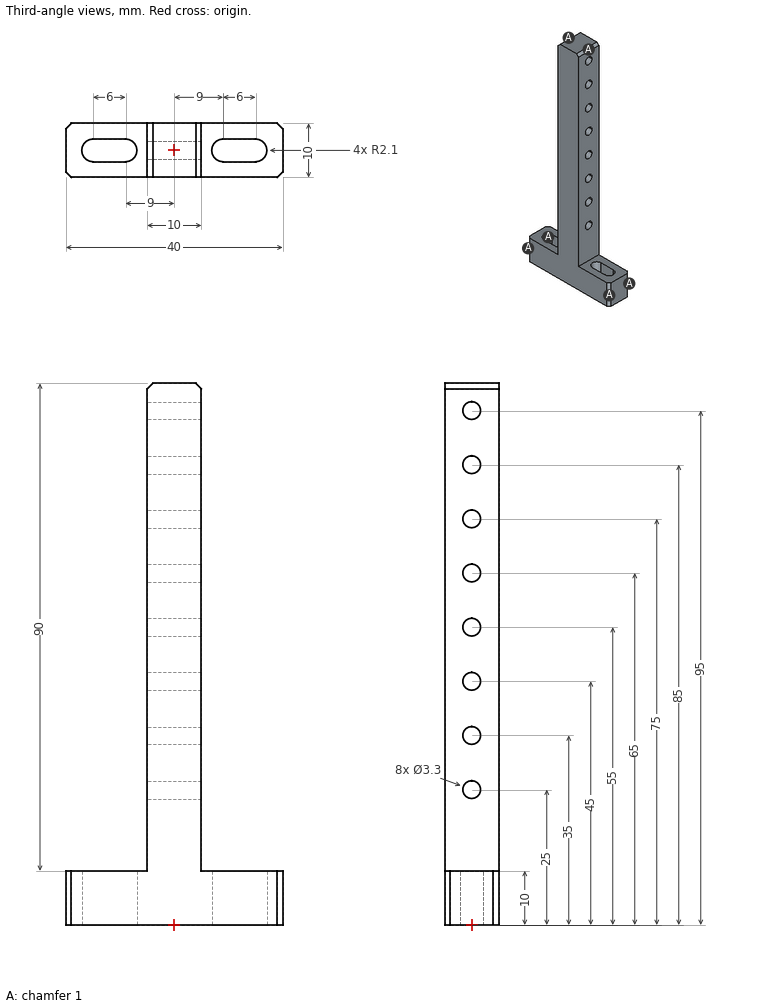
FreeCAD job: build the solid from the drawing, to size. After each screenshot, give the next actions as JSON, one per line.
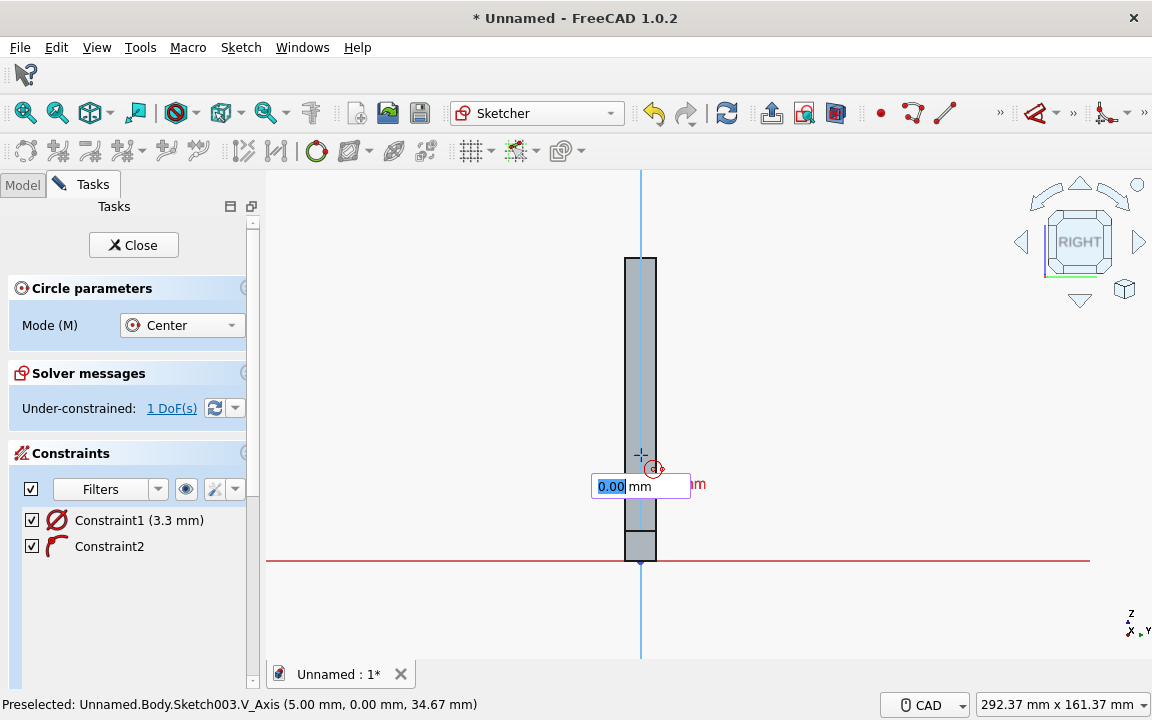
{"action": "scroll", "coordinate": [645, 453], "scroll_direction": "up", "scroll_amount": 7}
{"action": "mouse_move", "coordinate": [645, 452]}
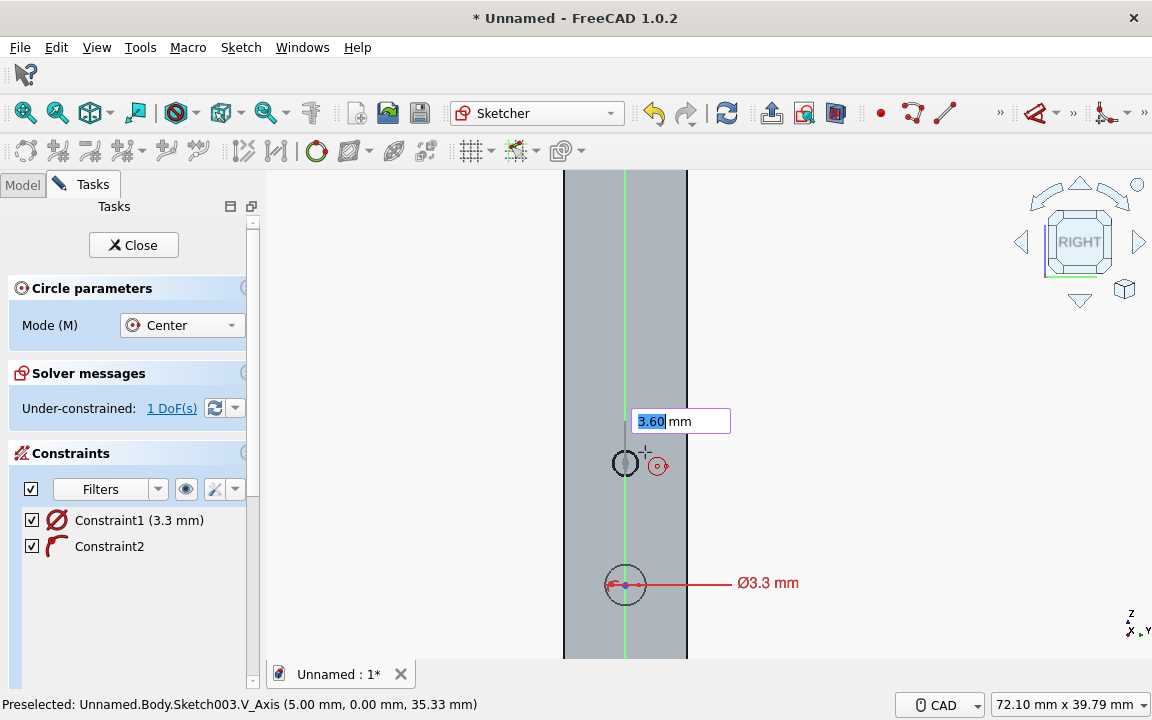
{"action": "type", "text": "3.3"}
{"action": "key", "text": "Return"}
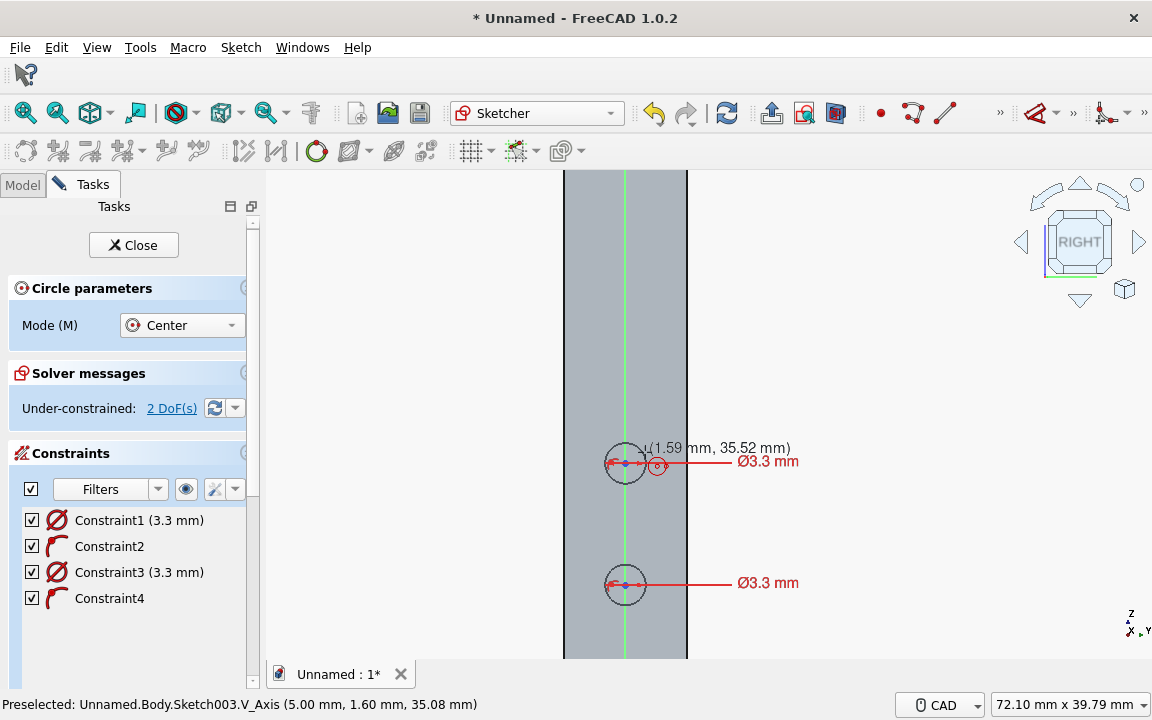
{"action": "scroll", "coordinate": [645, 453], "scroll_direction": "down", "scroll_amount": 7}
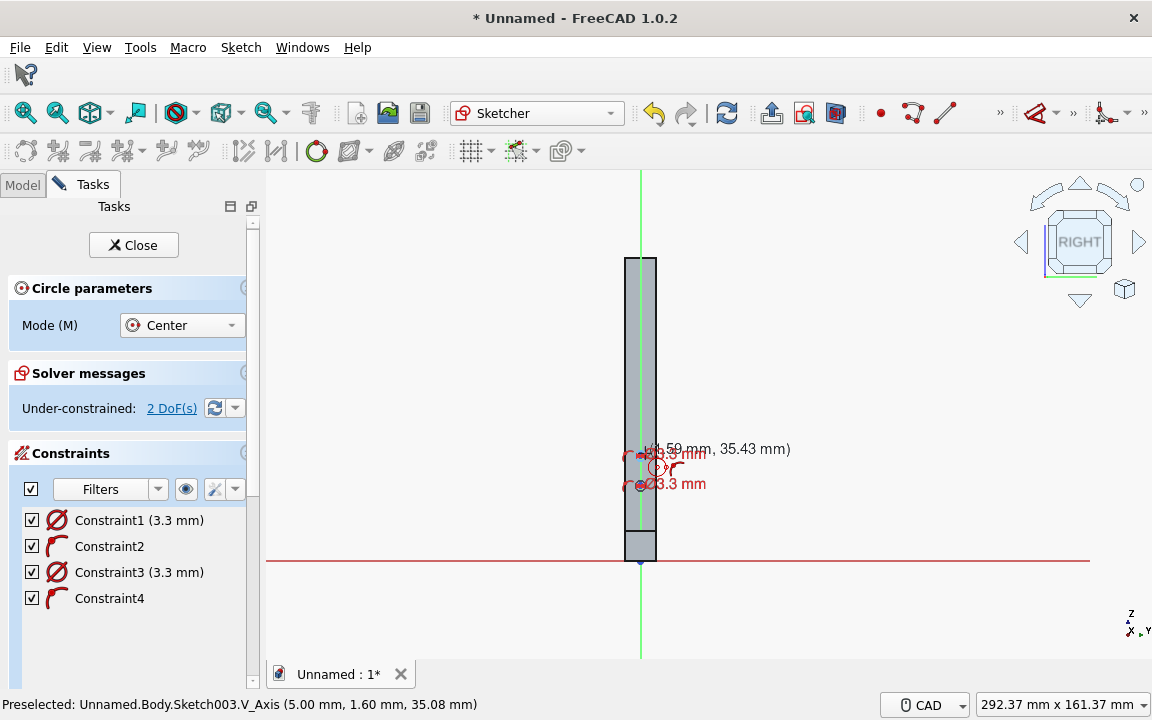
{"action": "left_click", "coordinate": [641, 425]}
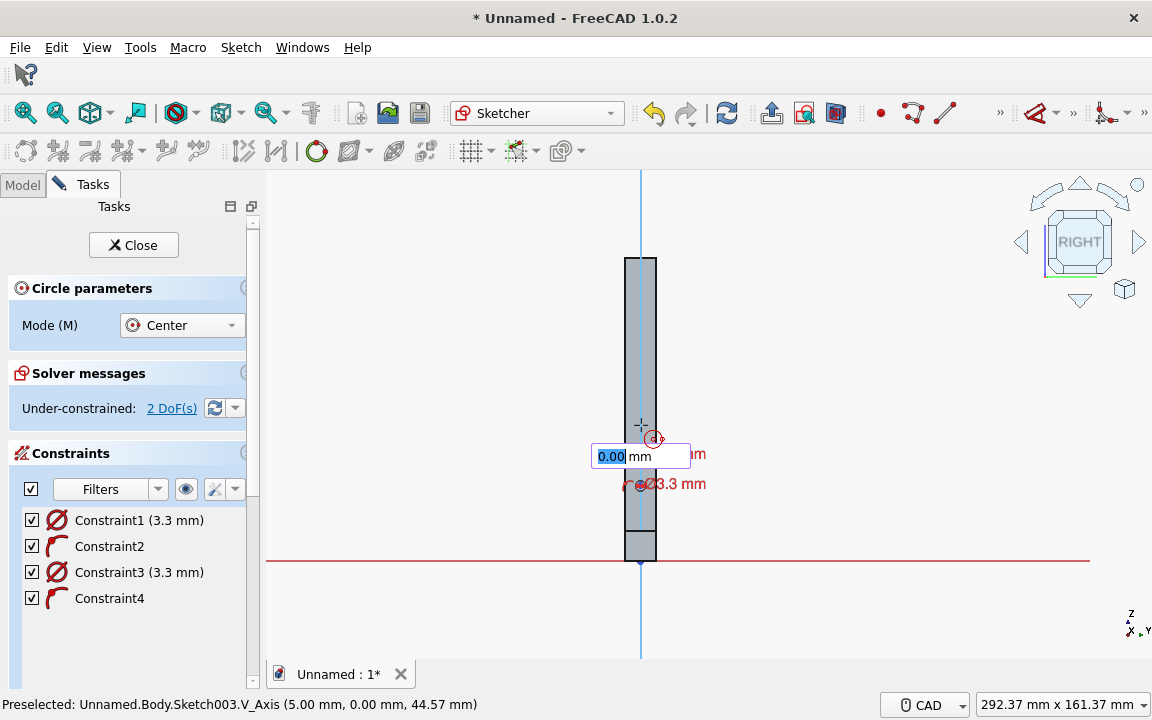
{"action": "scroll", "coordinate": [645, 423], "scroll_direction": "up", "scroll_amount": 7}
{"action": "mouse_move", "coordinate": [645, 421]}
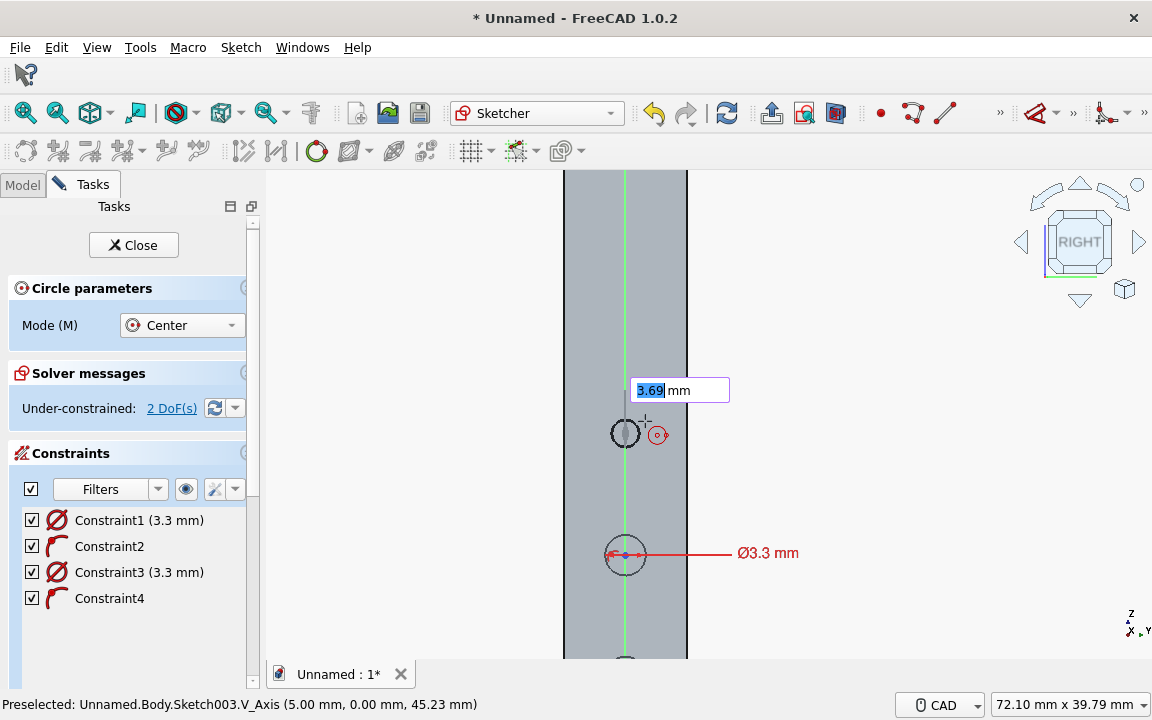
{"action": "type", "text": "3.3"}
{"action": "key", "text": "Return"}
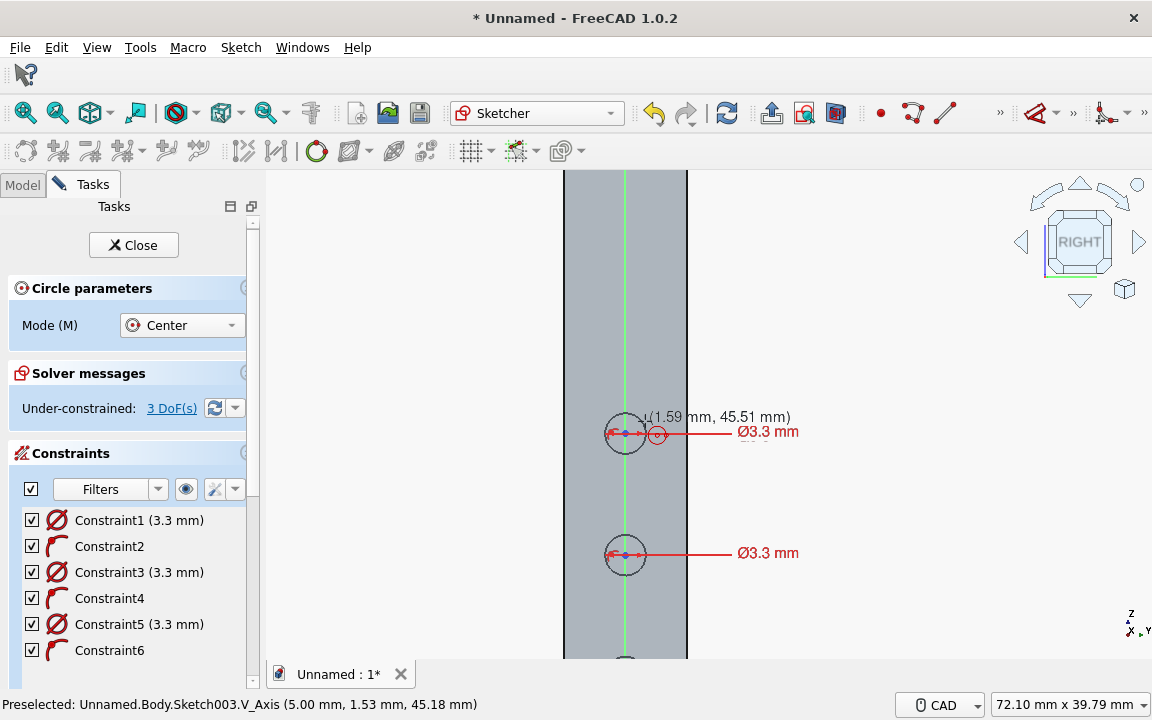
{"action": "scroll", "coordinate": [645, 423], "scroll_direction": "down", "scroll_amount": 7}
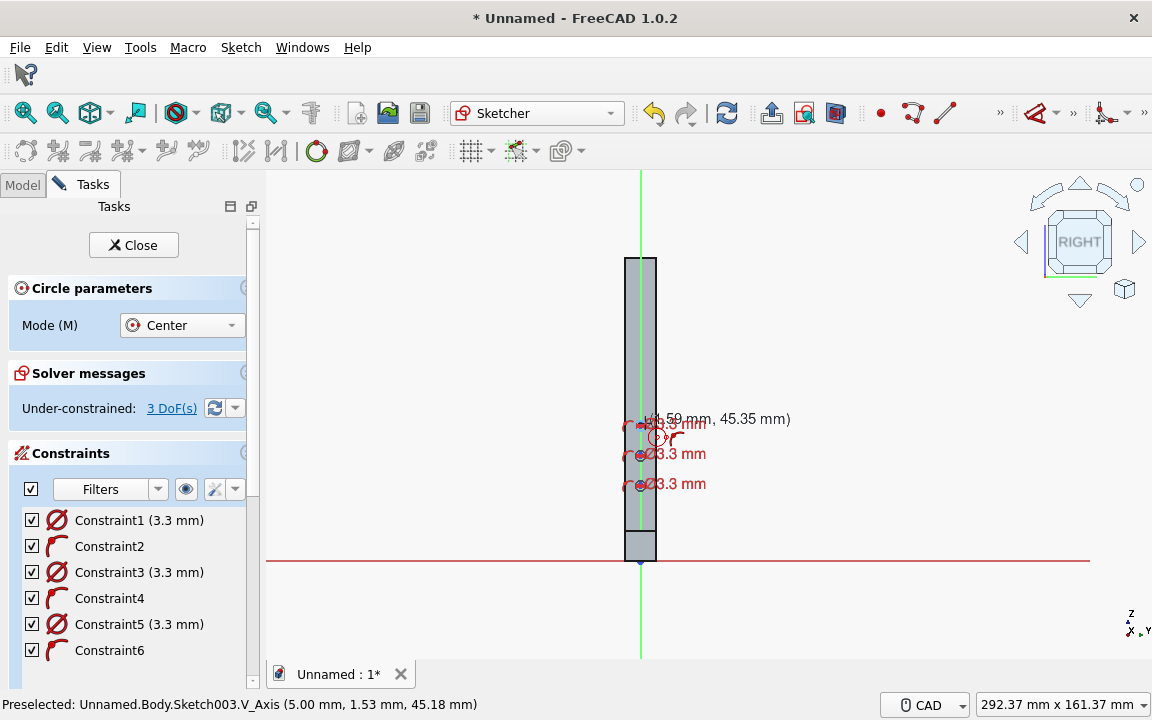
{"action": "left_click", "coordinate": [641, 394]}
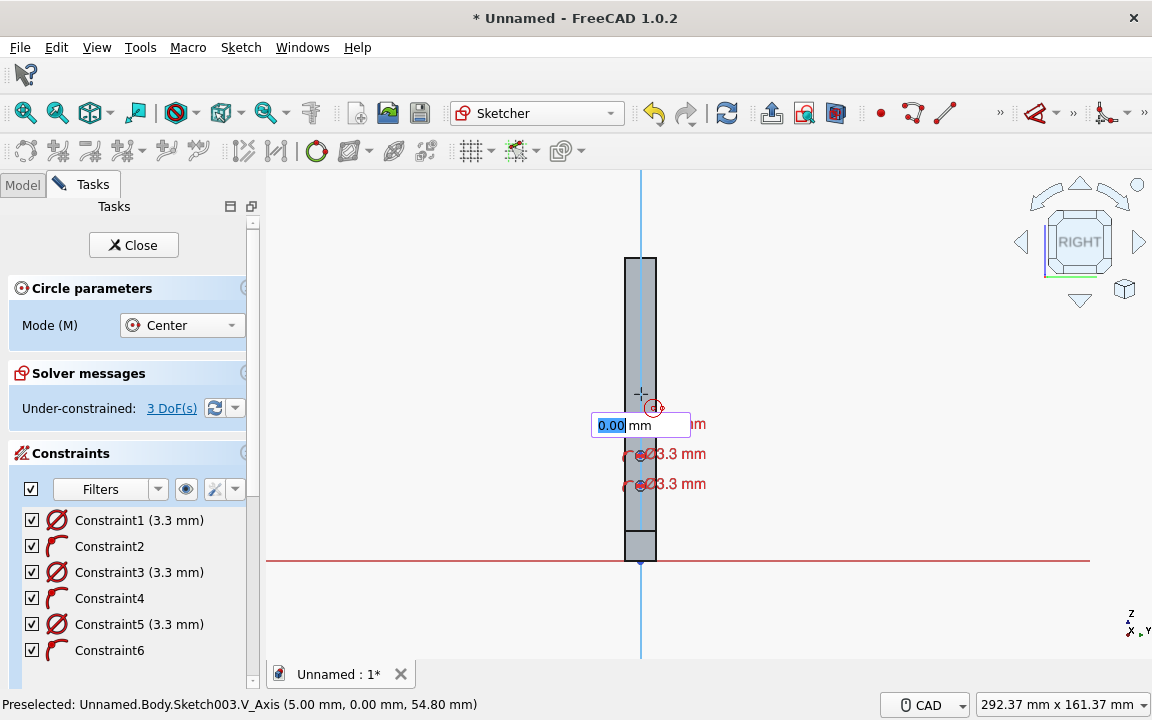
{"action": "scroll", "coordinate": [645, 393], "scroll_direction": "up", "scroll_amount": 7}
{"action": "mouse_move", "coordinate": [645, 390]}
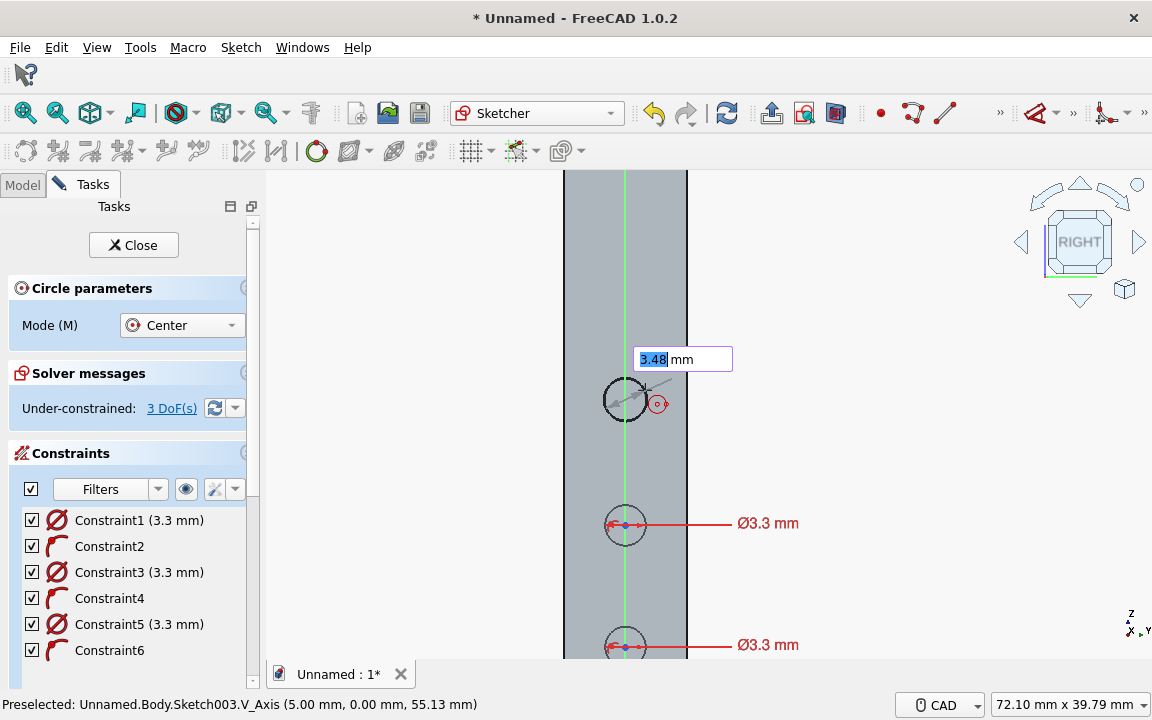
{"action": "type", "text": "3.3"}
{"action": "key", "text": "Return"}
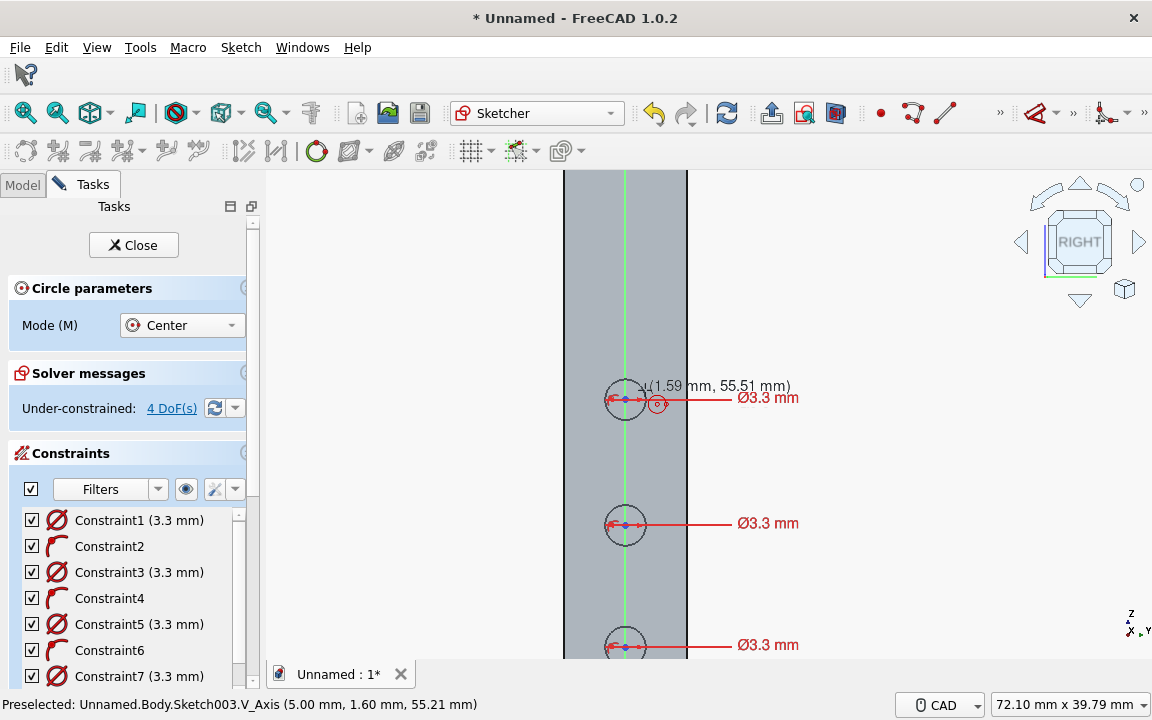
{"action": "scroll", "coordinate": [645, 393], "scroll_direction": "down", "scroll_amount": 7}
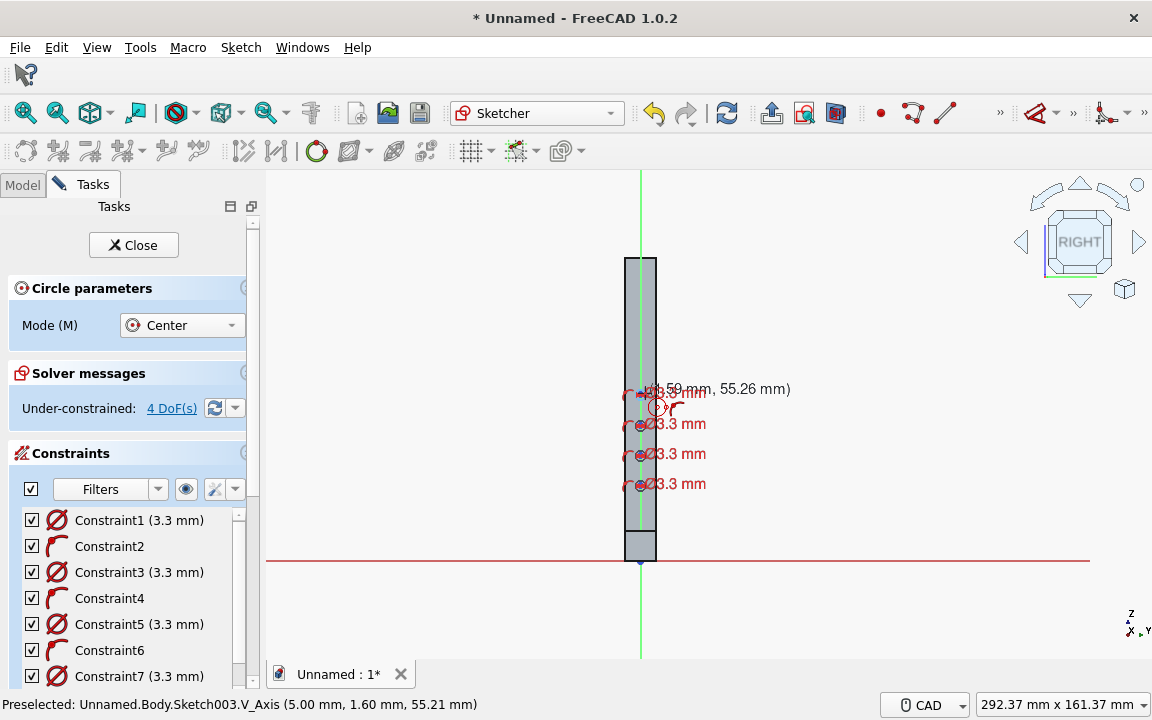
{"action": "left_click", "coordinate": [641, 364]}